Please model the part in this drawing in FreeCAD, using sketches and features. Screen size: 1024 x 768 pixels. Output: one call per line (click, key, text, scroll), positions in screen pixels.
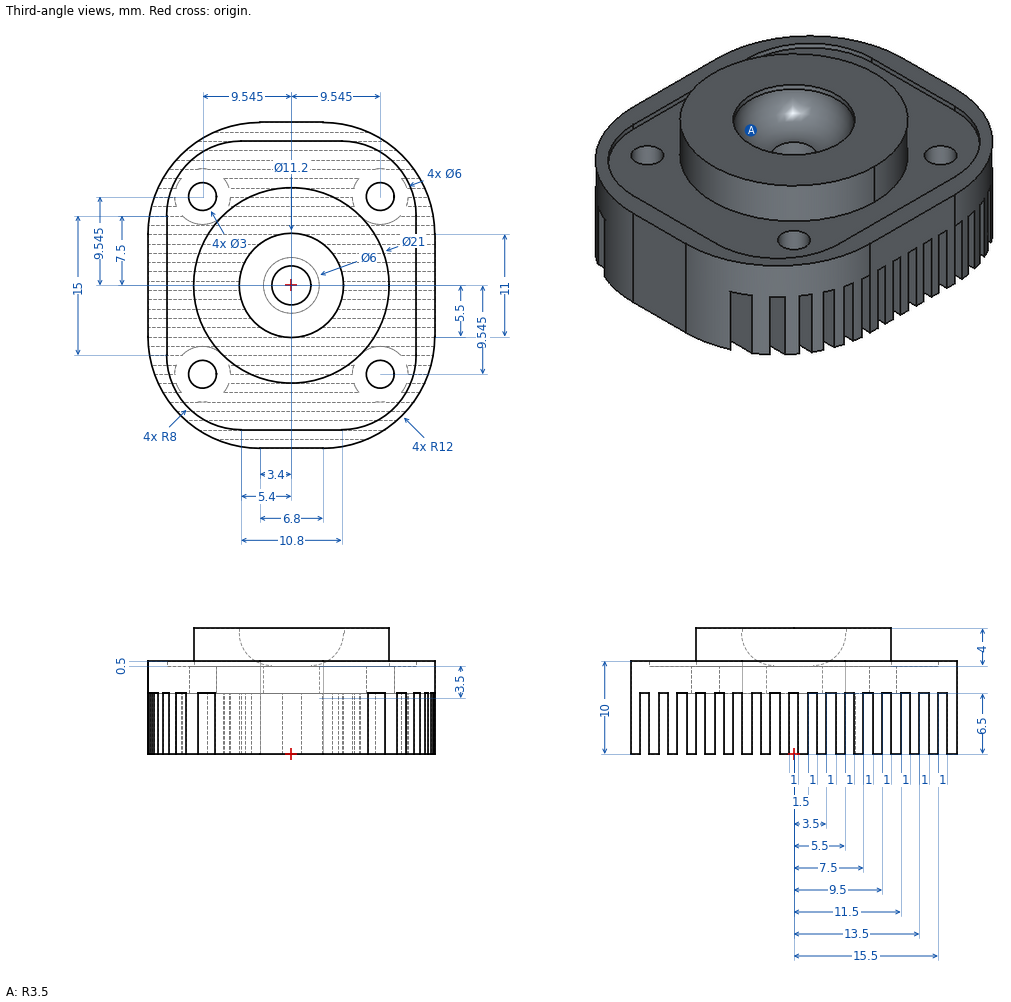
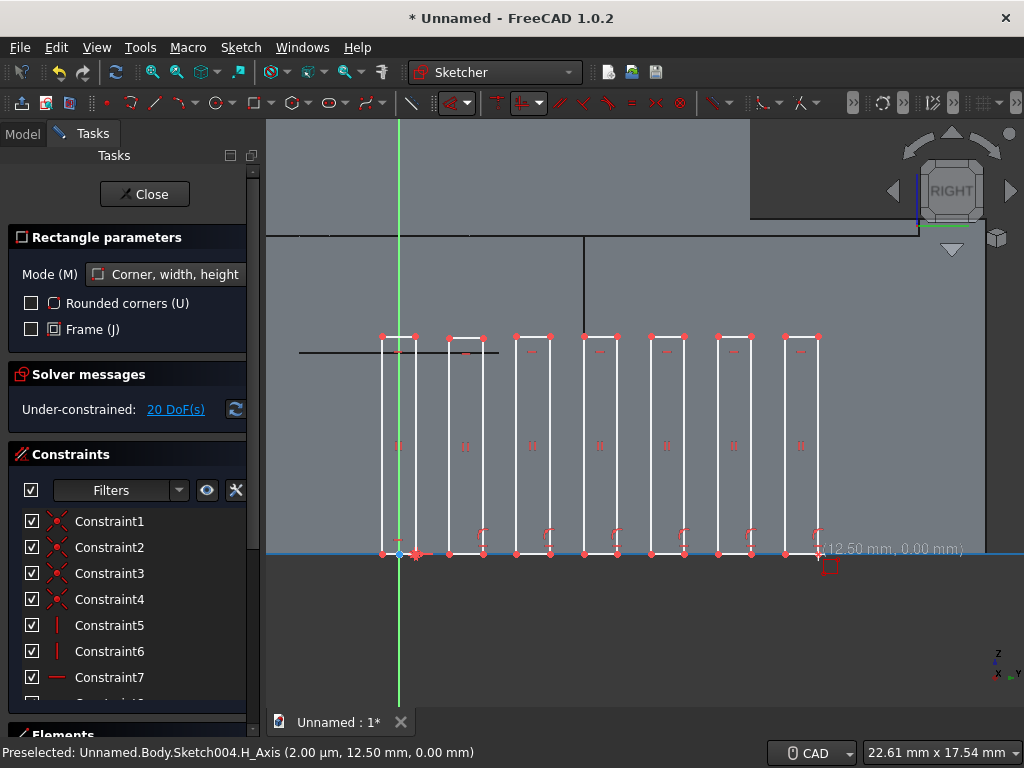
click(852, 336)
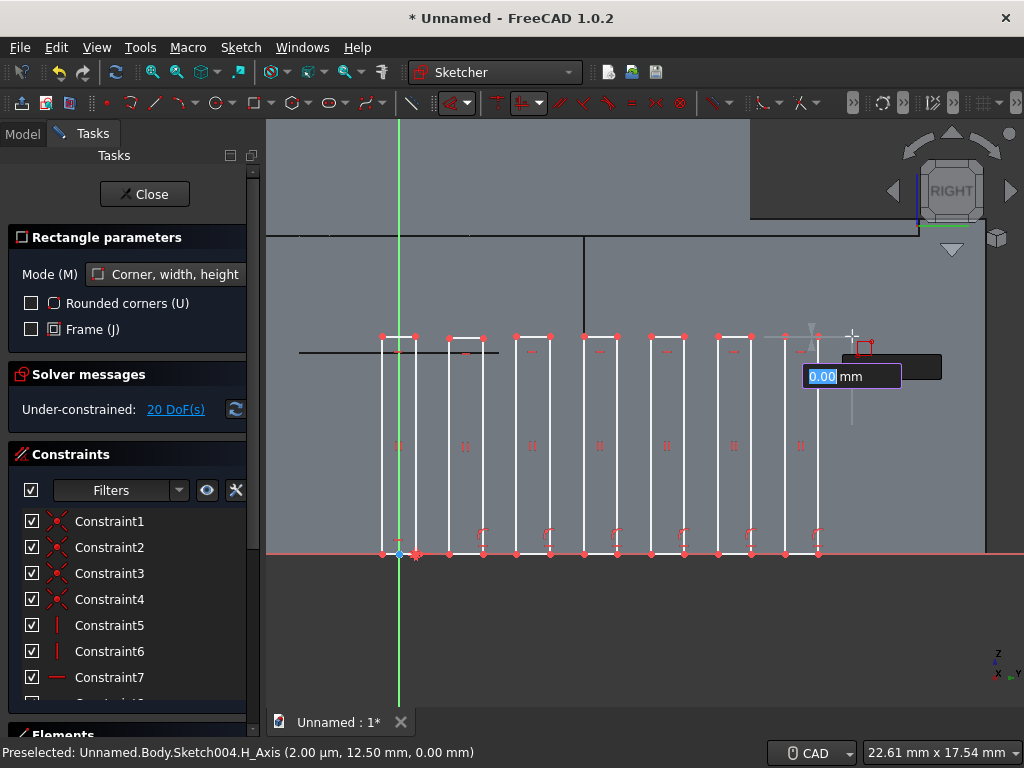
scroll(392, 348, down, 2)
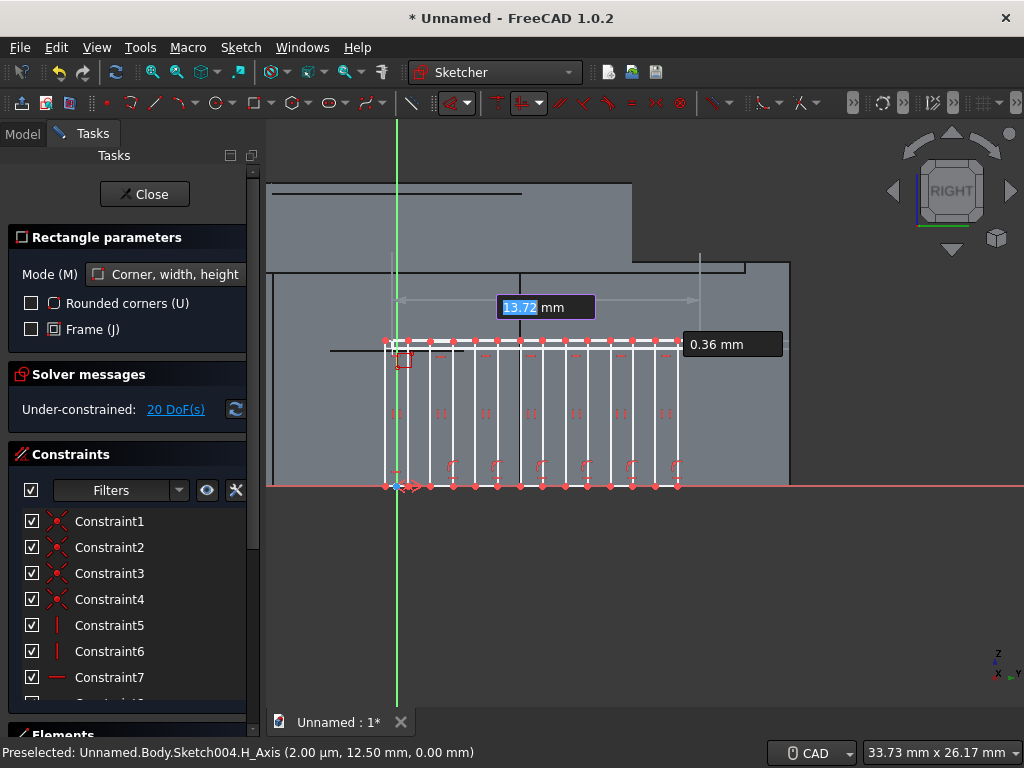
click(723, 486)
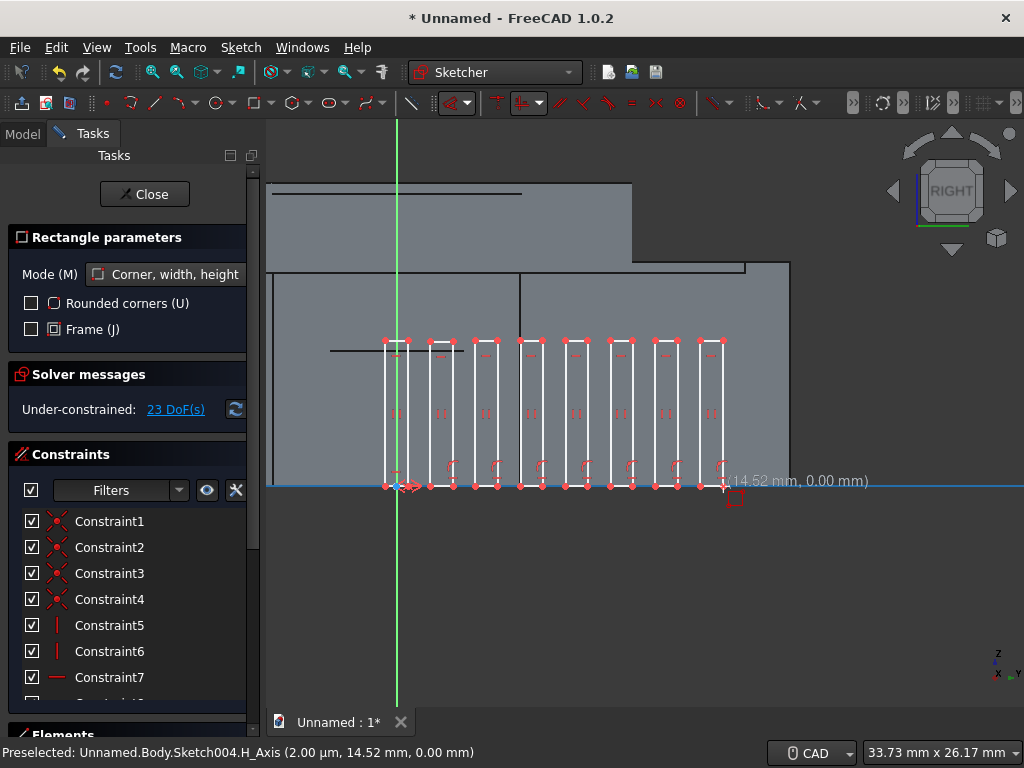
click(745, 340)
click(768, 486)
key(Escape)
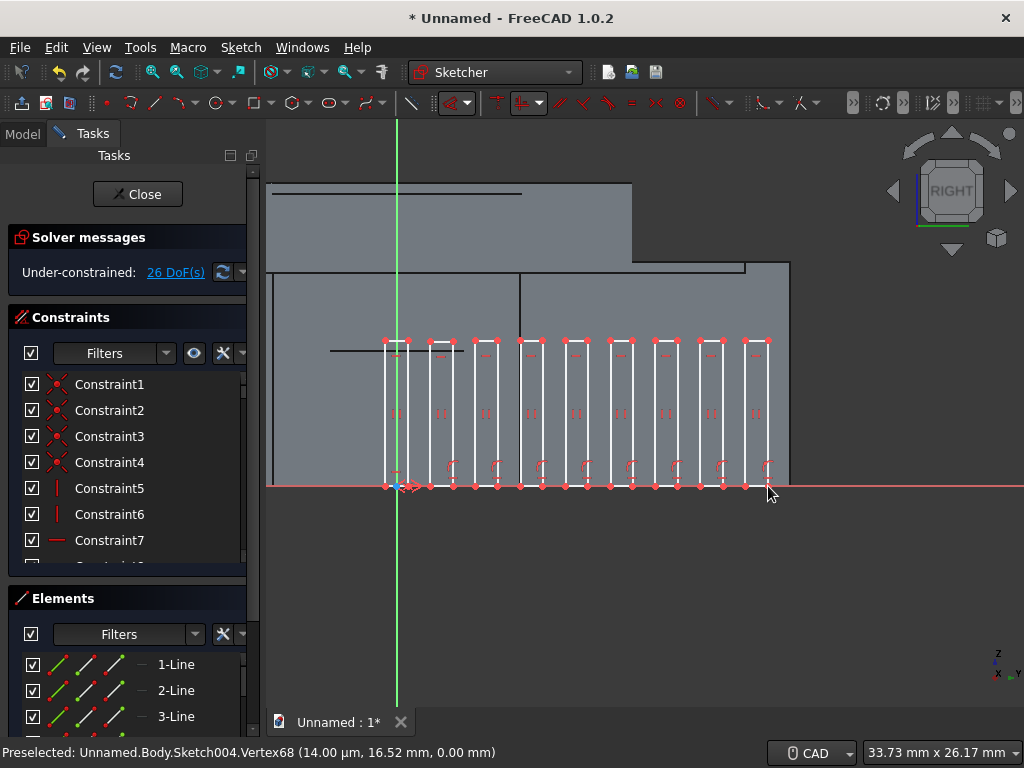
scroll(440, 486, up, 3)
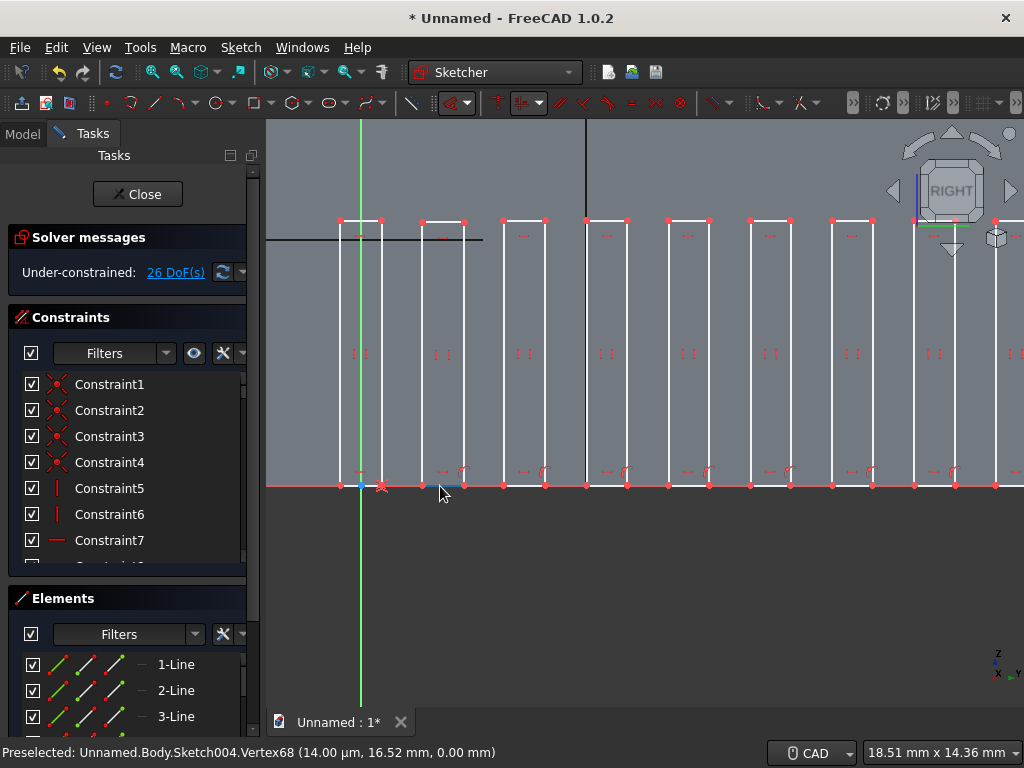
click(439, 486)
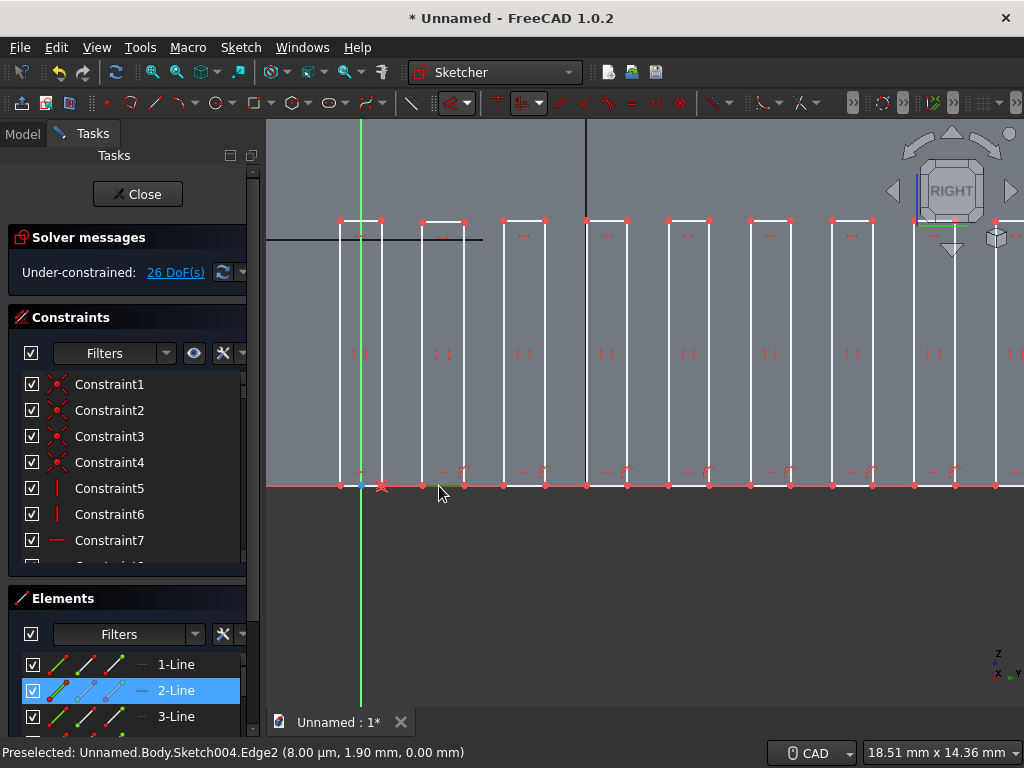
key(l)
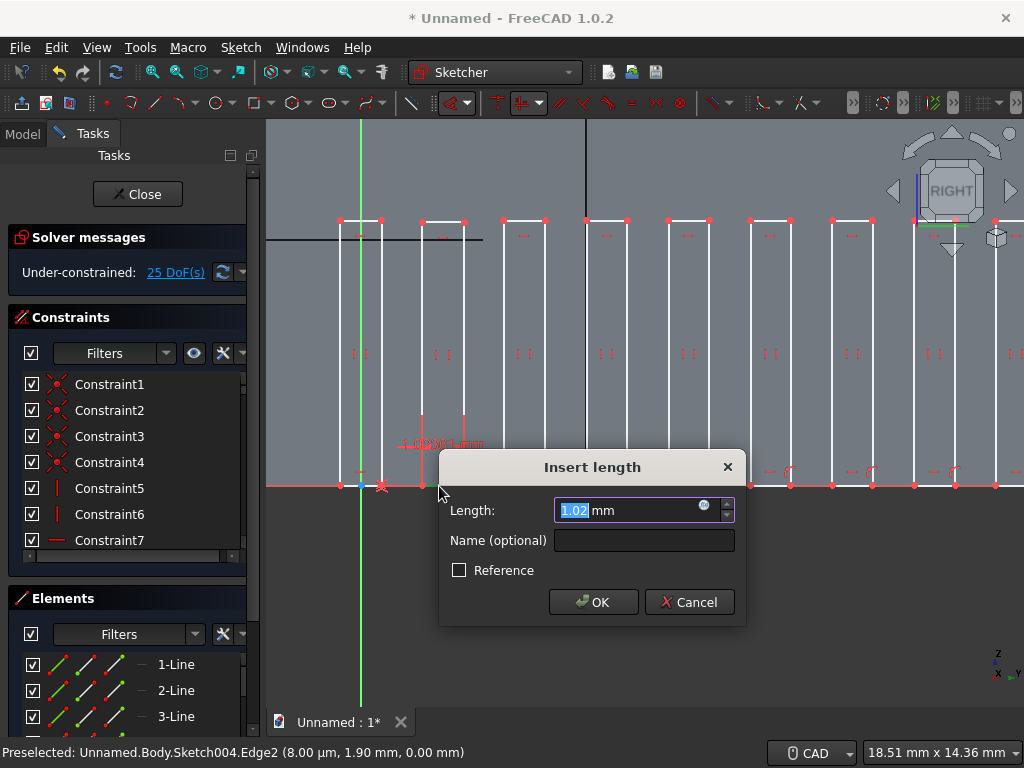
text(1)
key(Return)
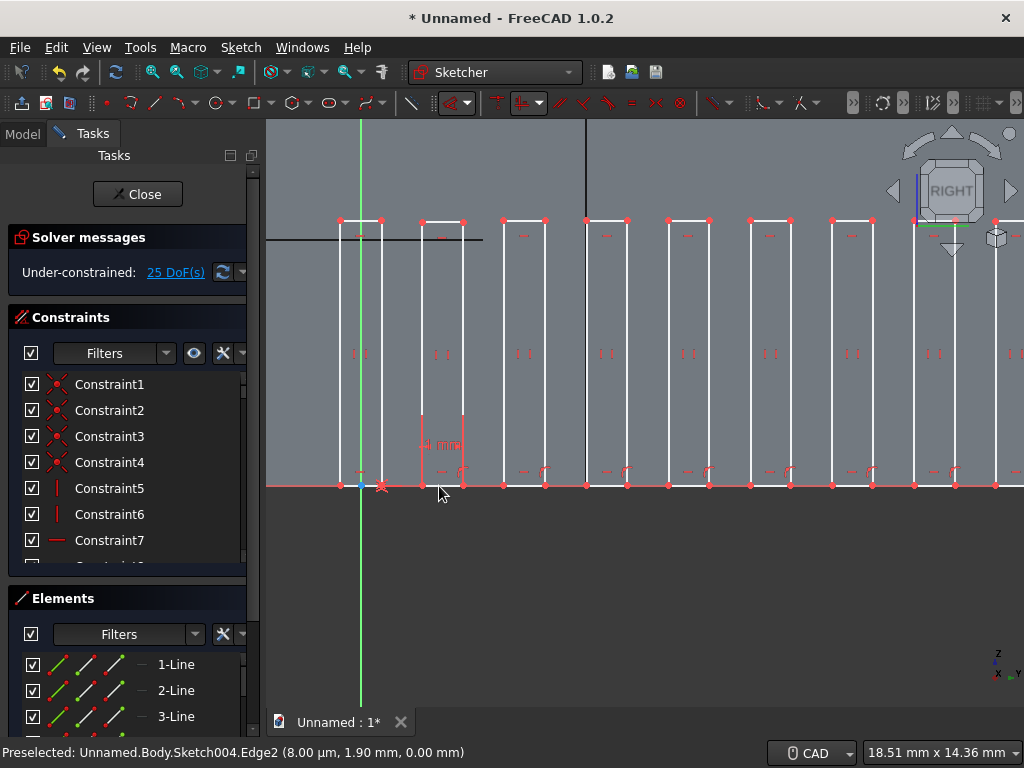
click(353, 486)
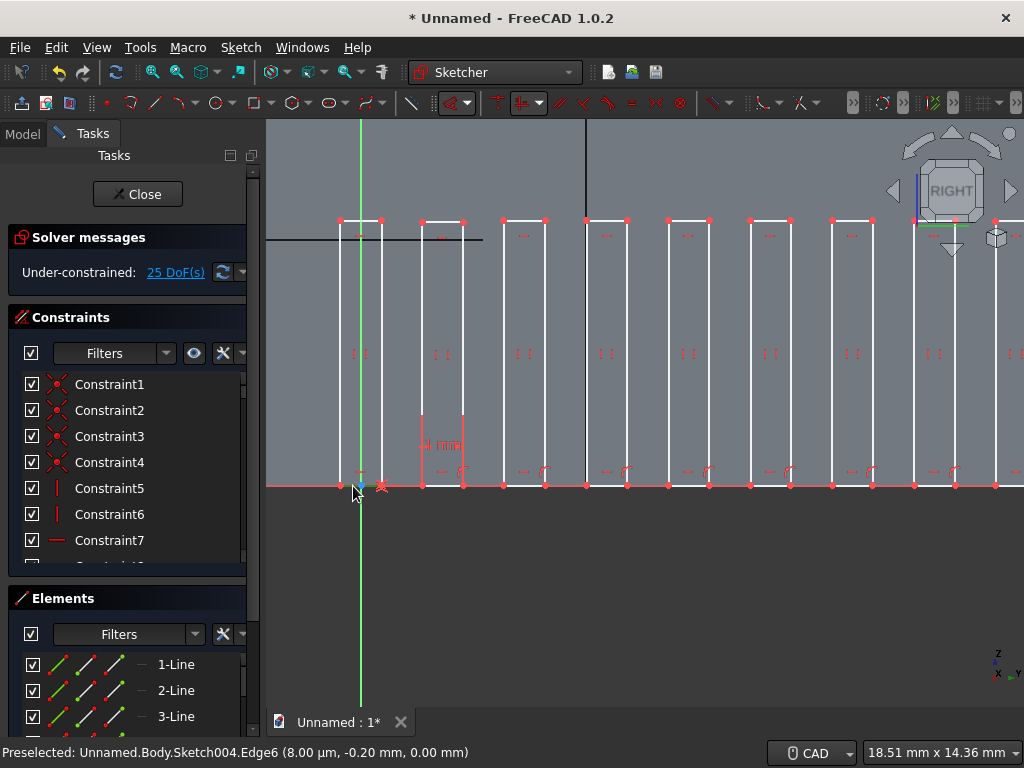
key(l)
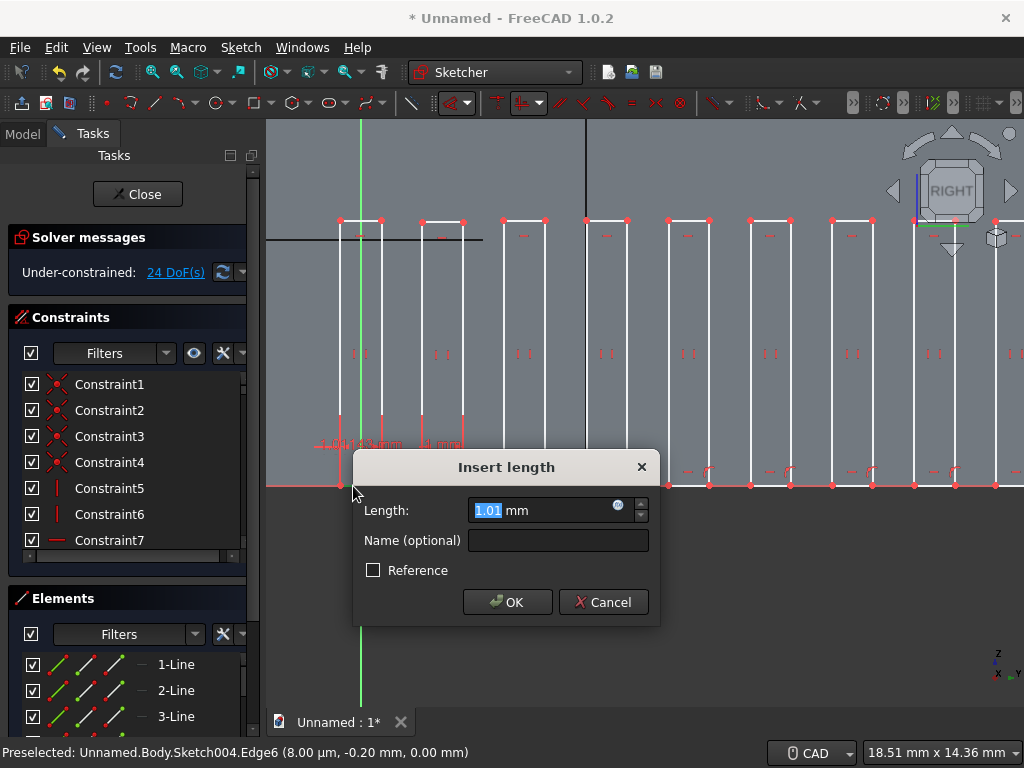
text(1)
key(Return)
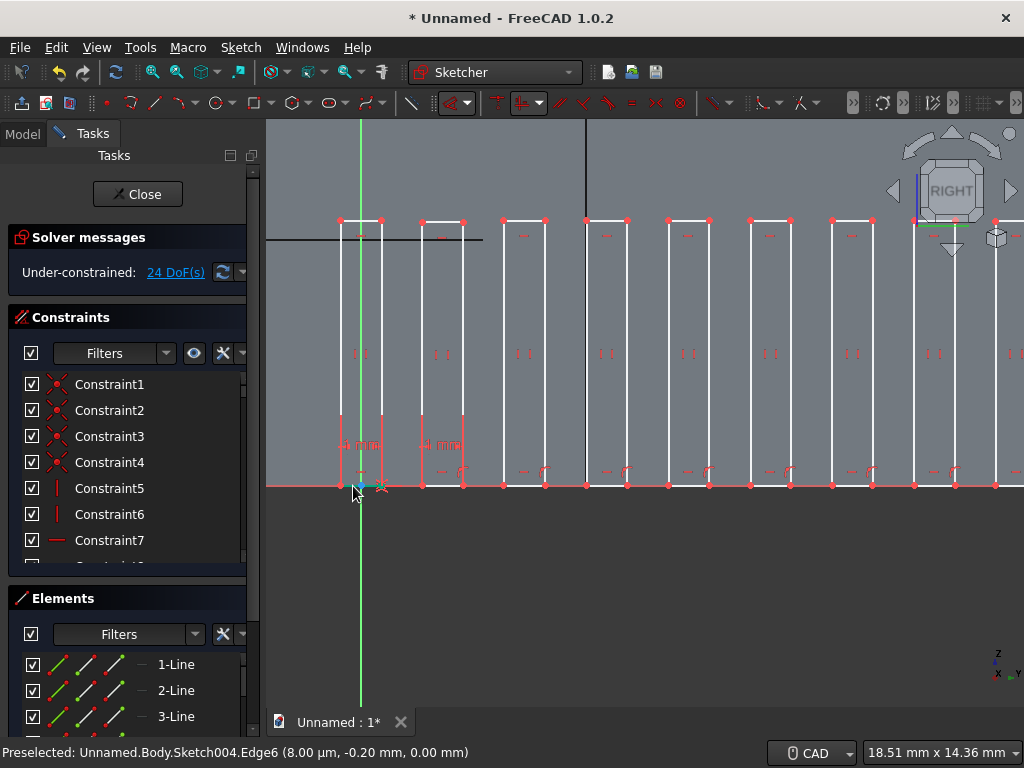
click(516, 486)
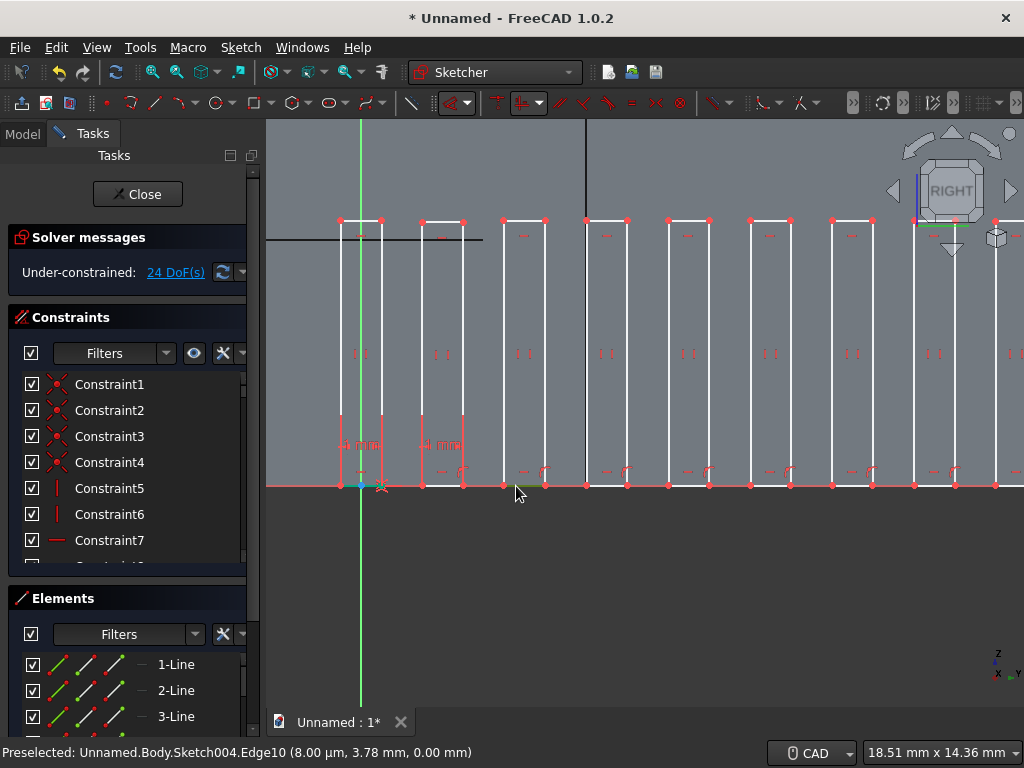
key(l)